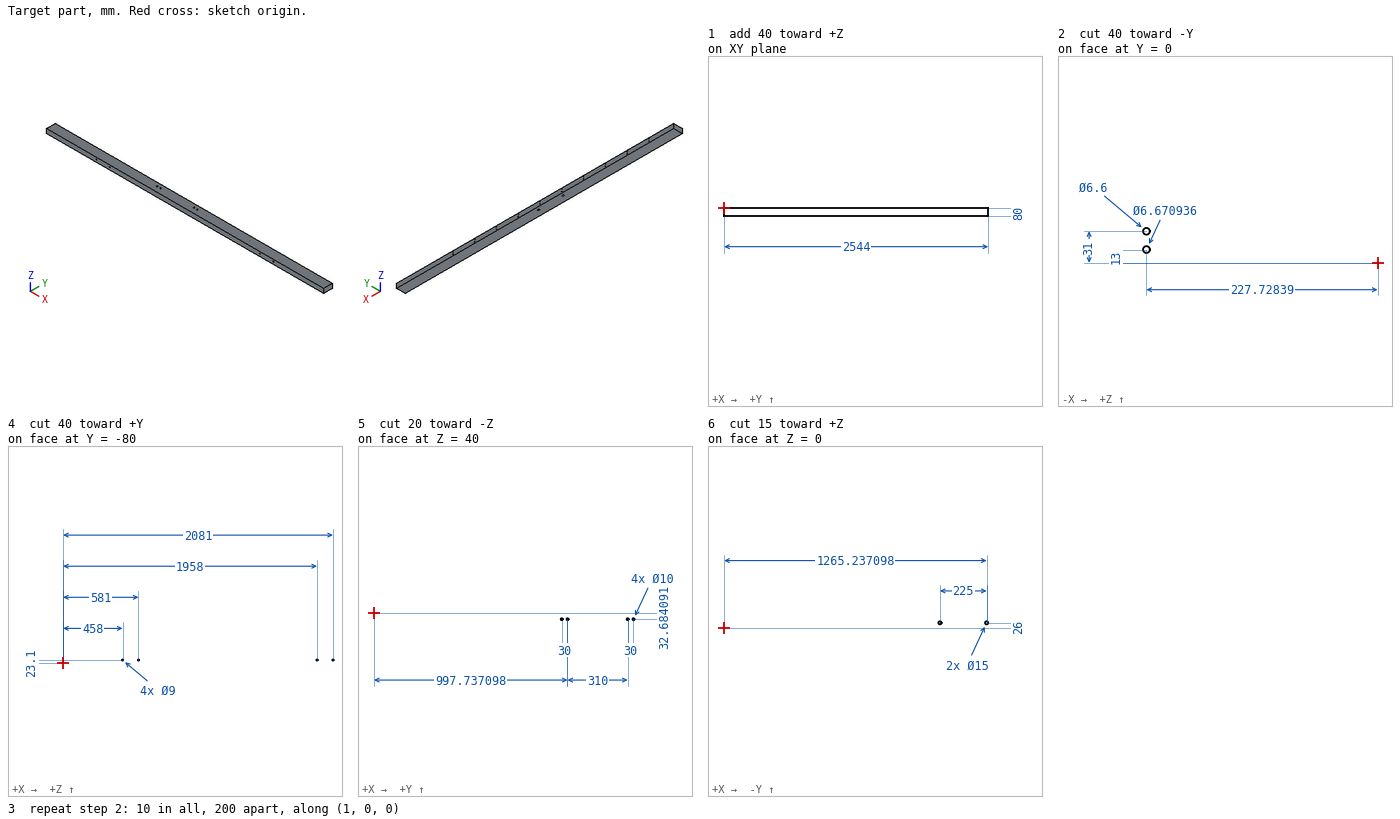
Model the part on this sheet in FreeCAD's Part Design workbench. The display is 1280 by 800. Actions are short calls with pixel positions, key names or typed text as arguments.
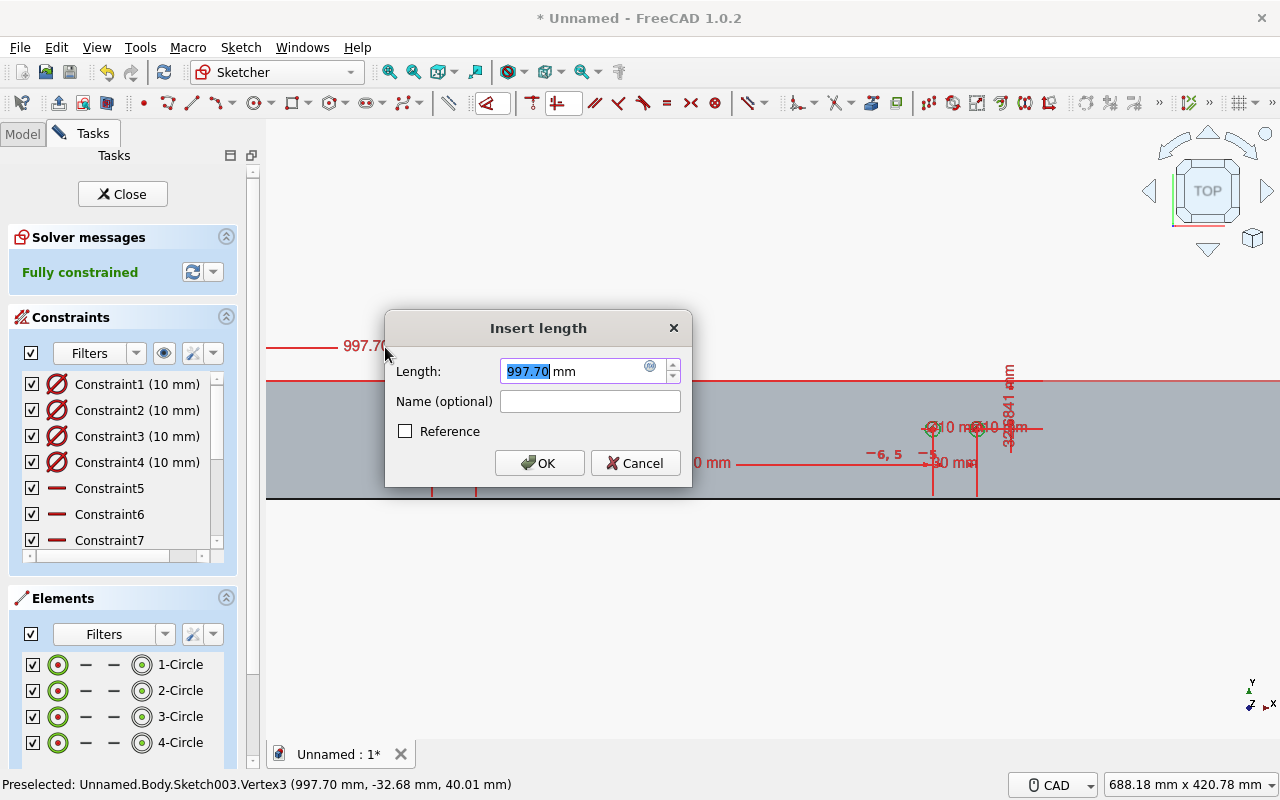
text(997.737098)
key(Return)
key(Escape)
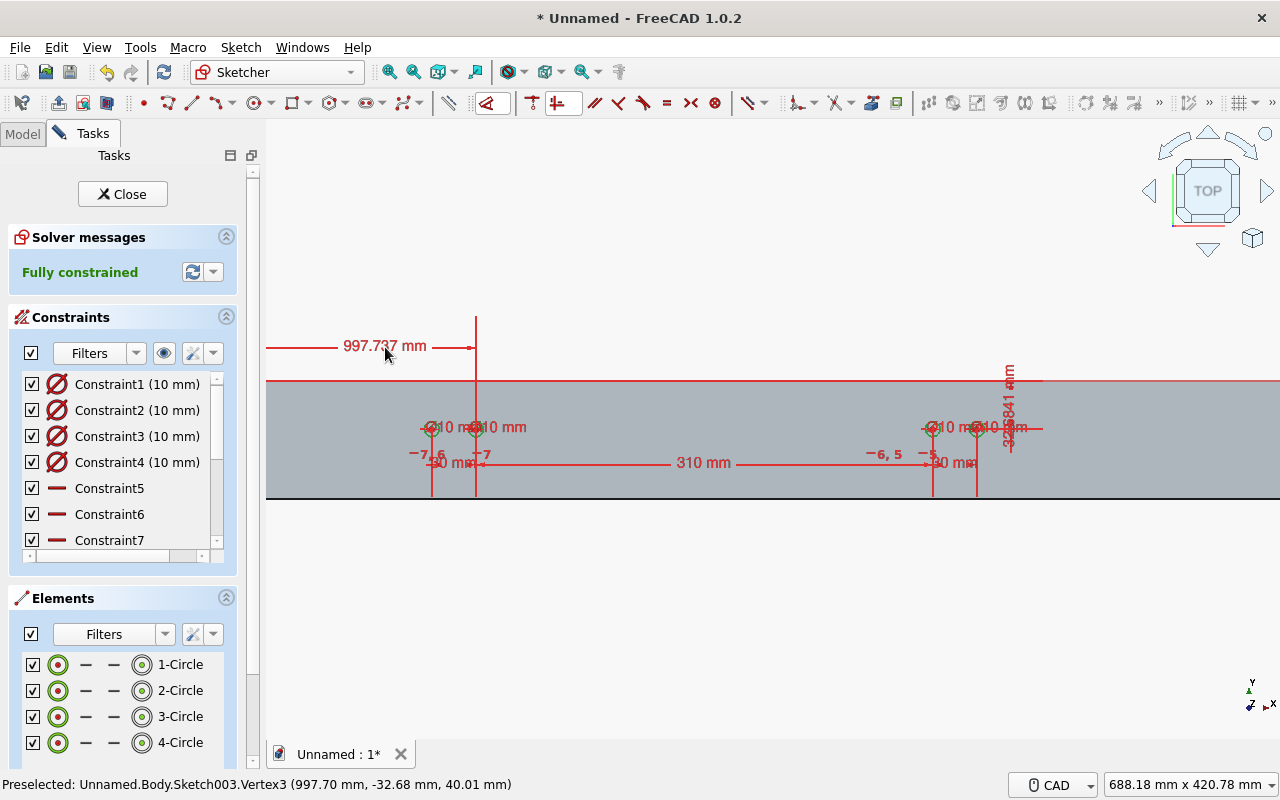
click(123, 194)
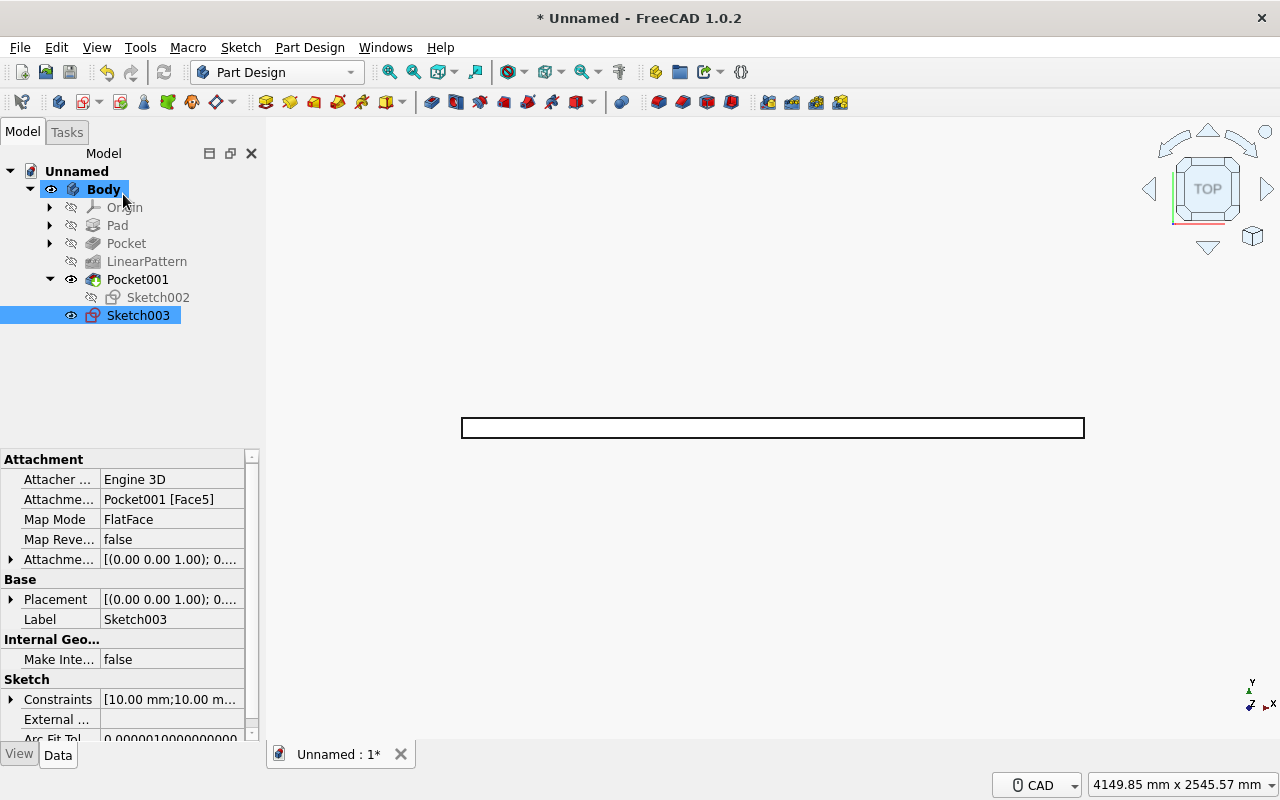
click(432, 102)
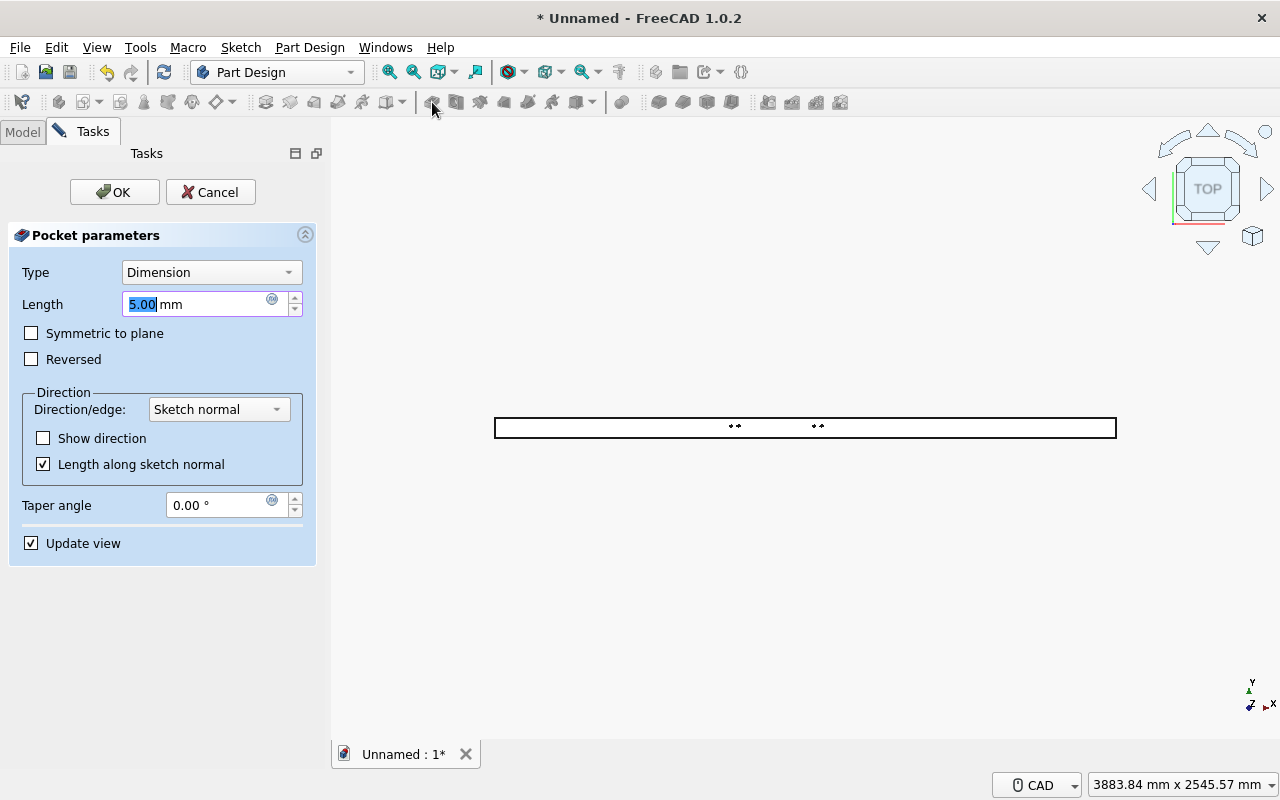
text(20)
key(Tab)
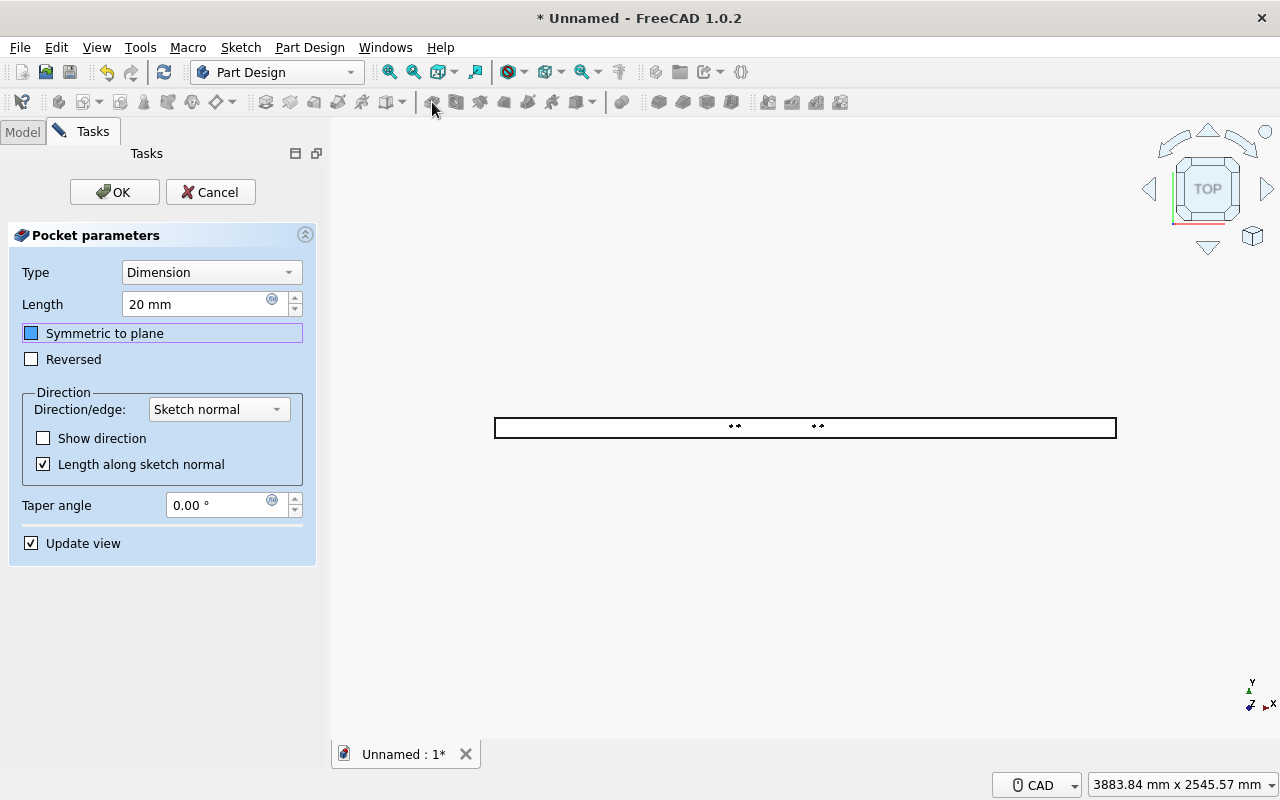
click(115, 192)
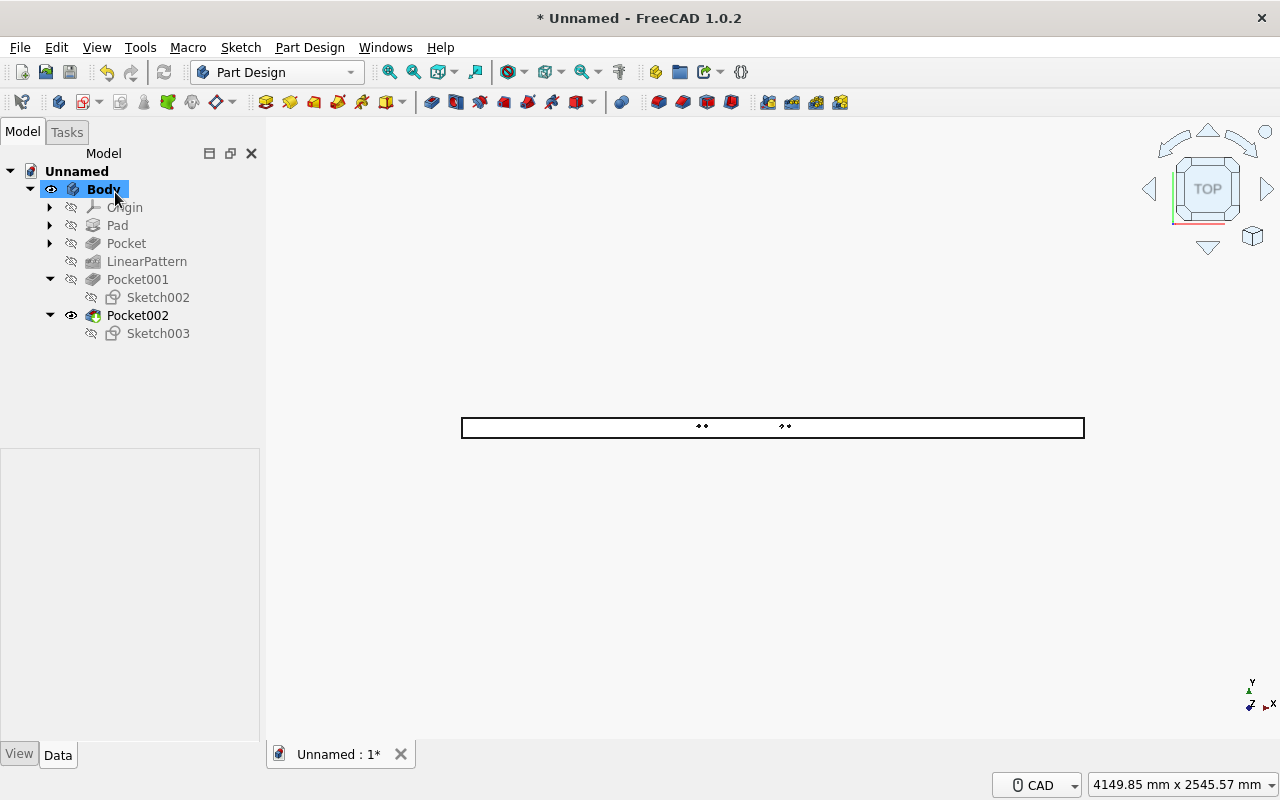
key(5)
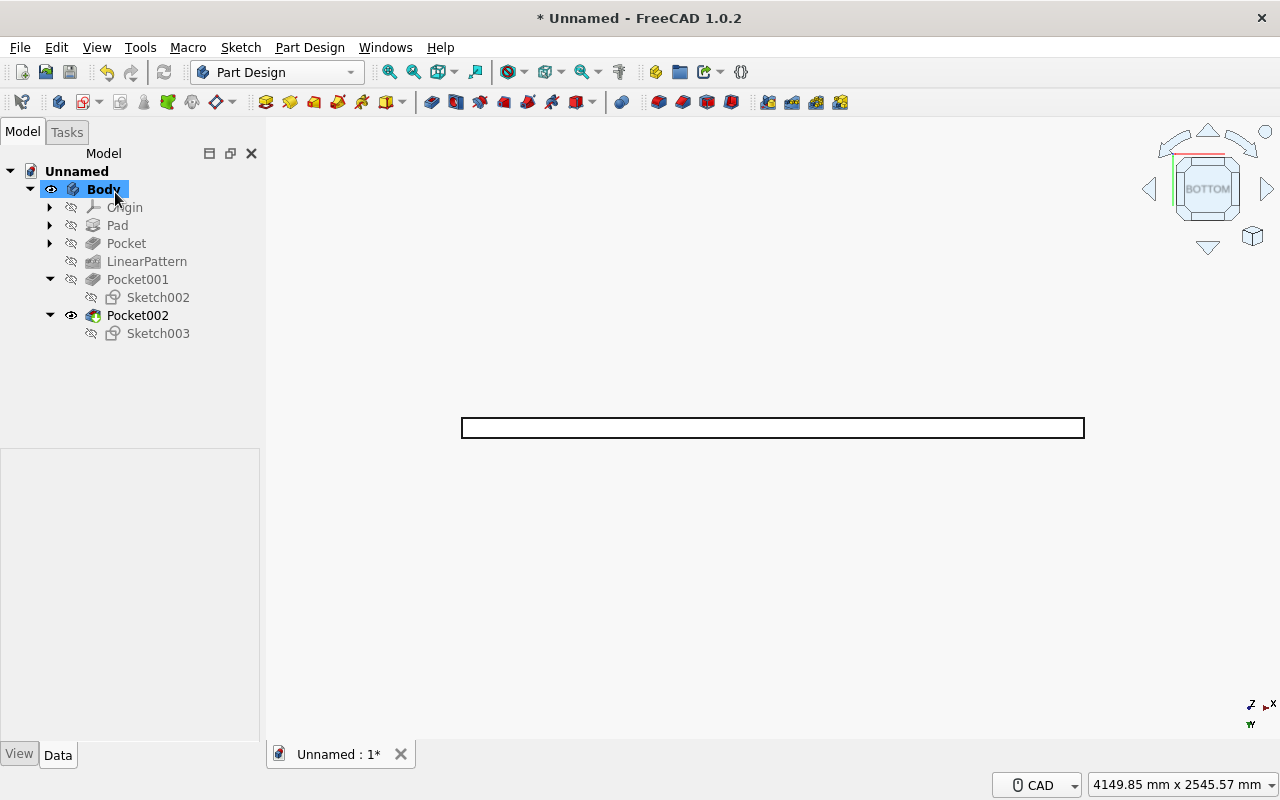
click(1039, 427)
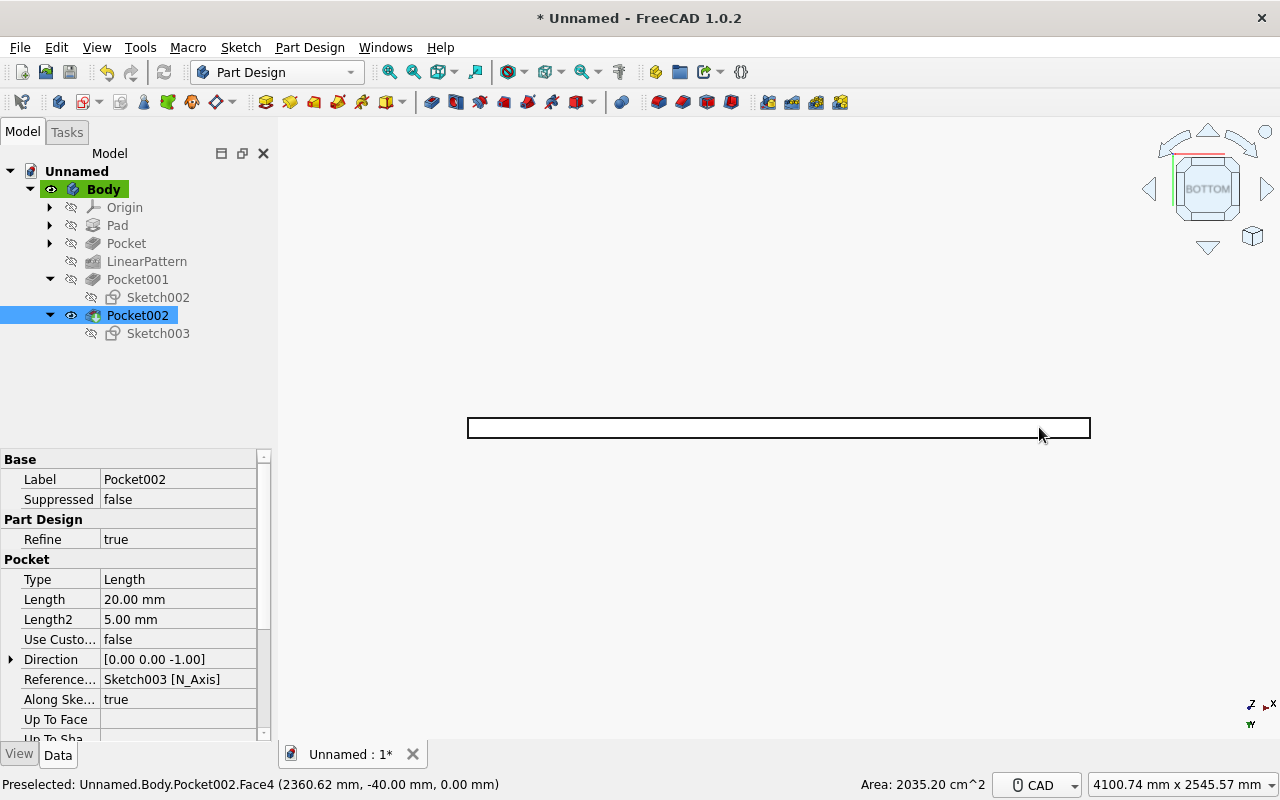
click(84, 102)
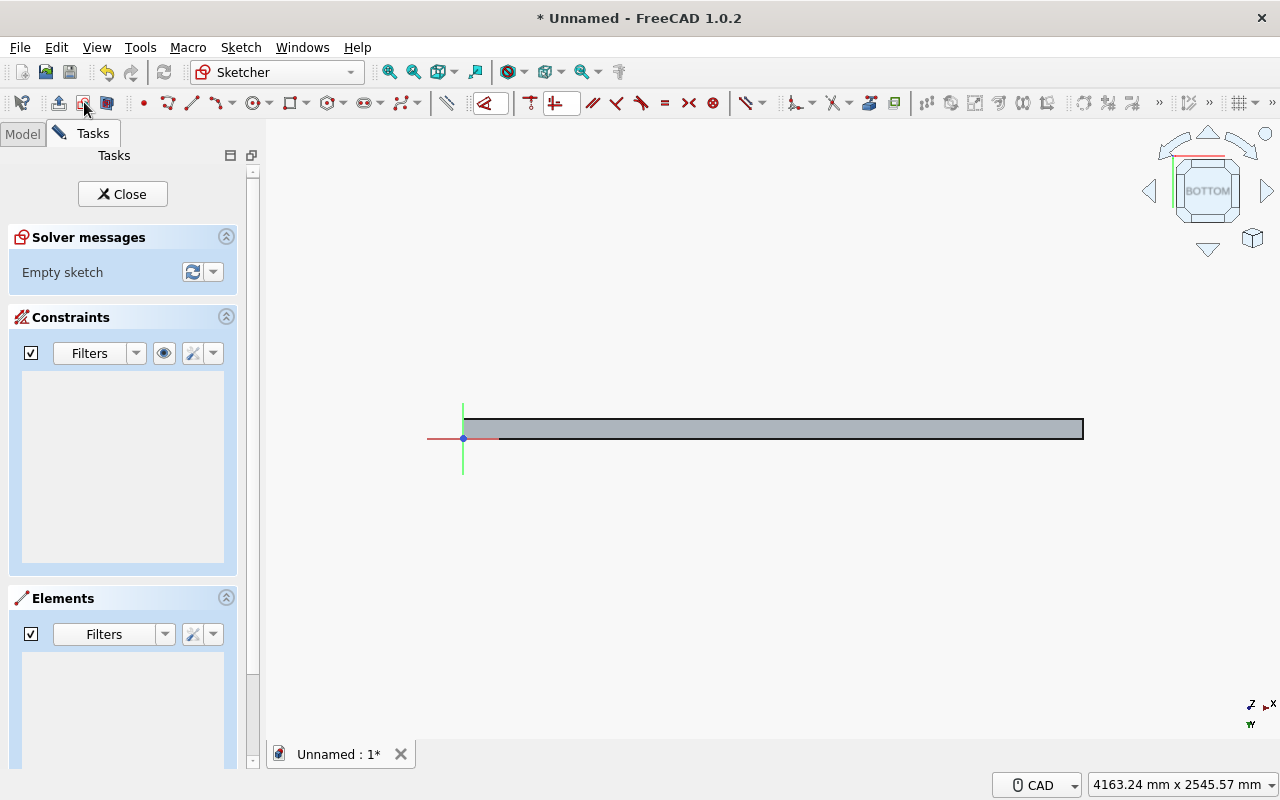
scroll(749, 433, up, 11)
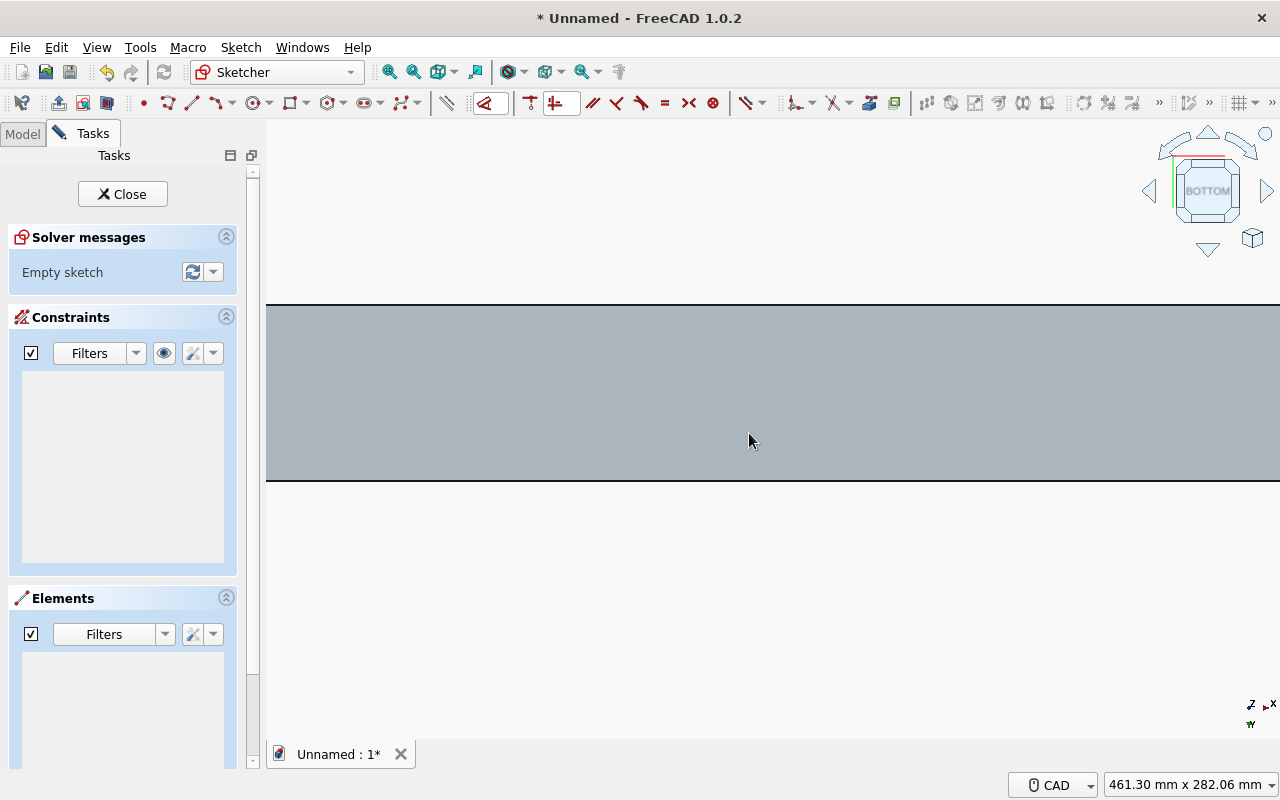
key(g)
key(c)